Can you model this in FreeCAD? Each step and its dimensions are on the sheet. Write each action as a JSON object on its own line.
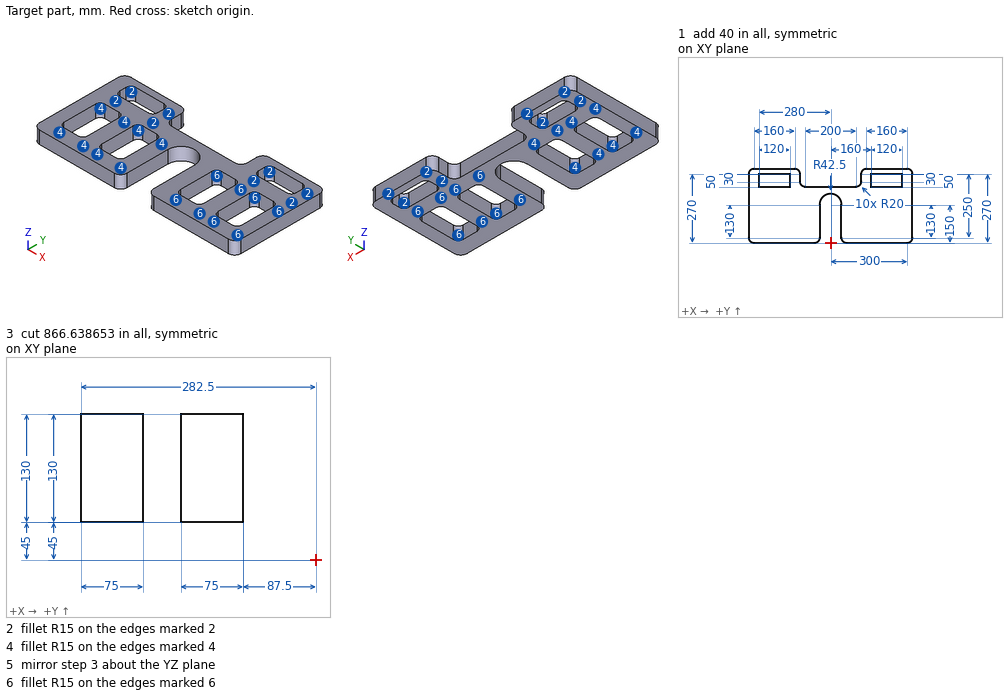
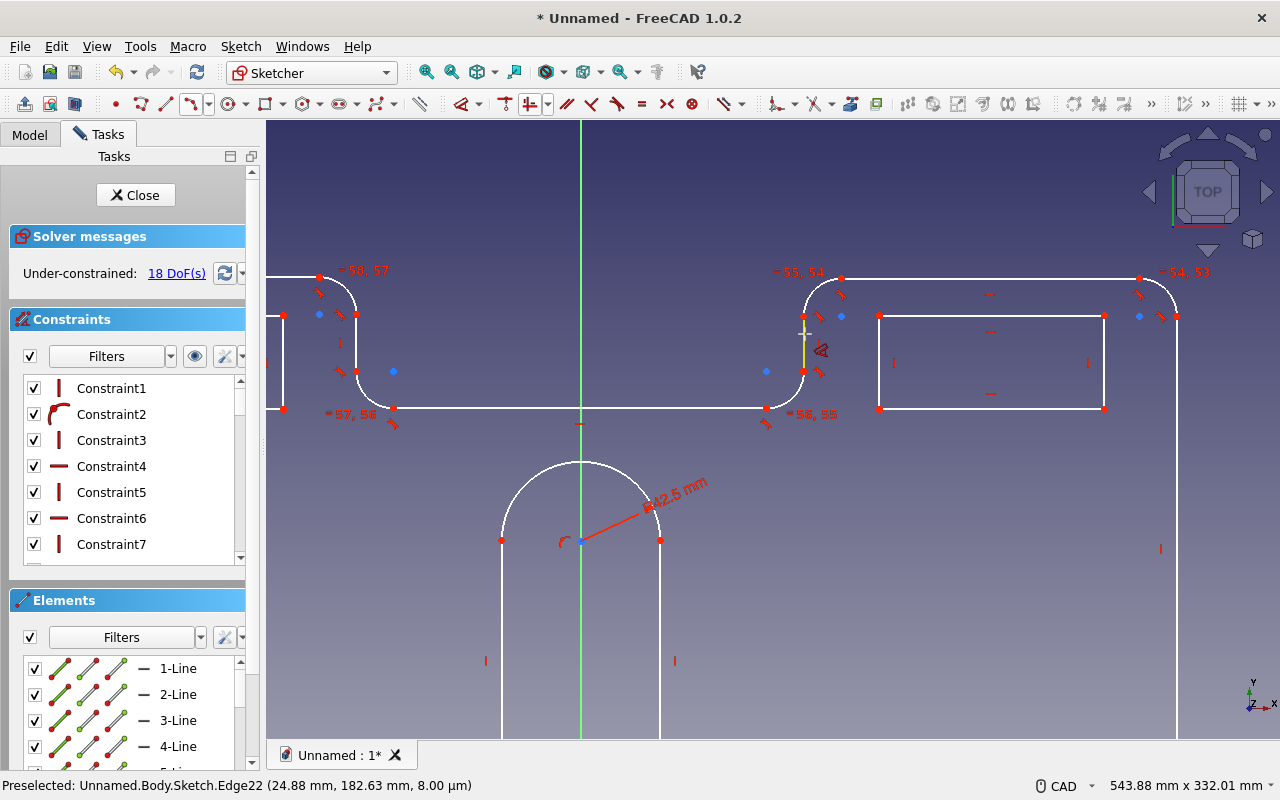
{"action": "left_click", "coordinate": [804, 333]}
{"action": "left_click", "coordinate": [838, 344]}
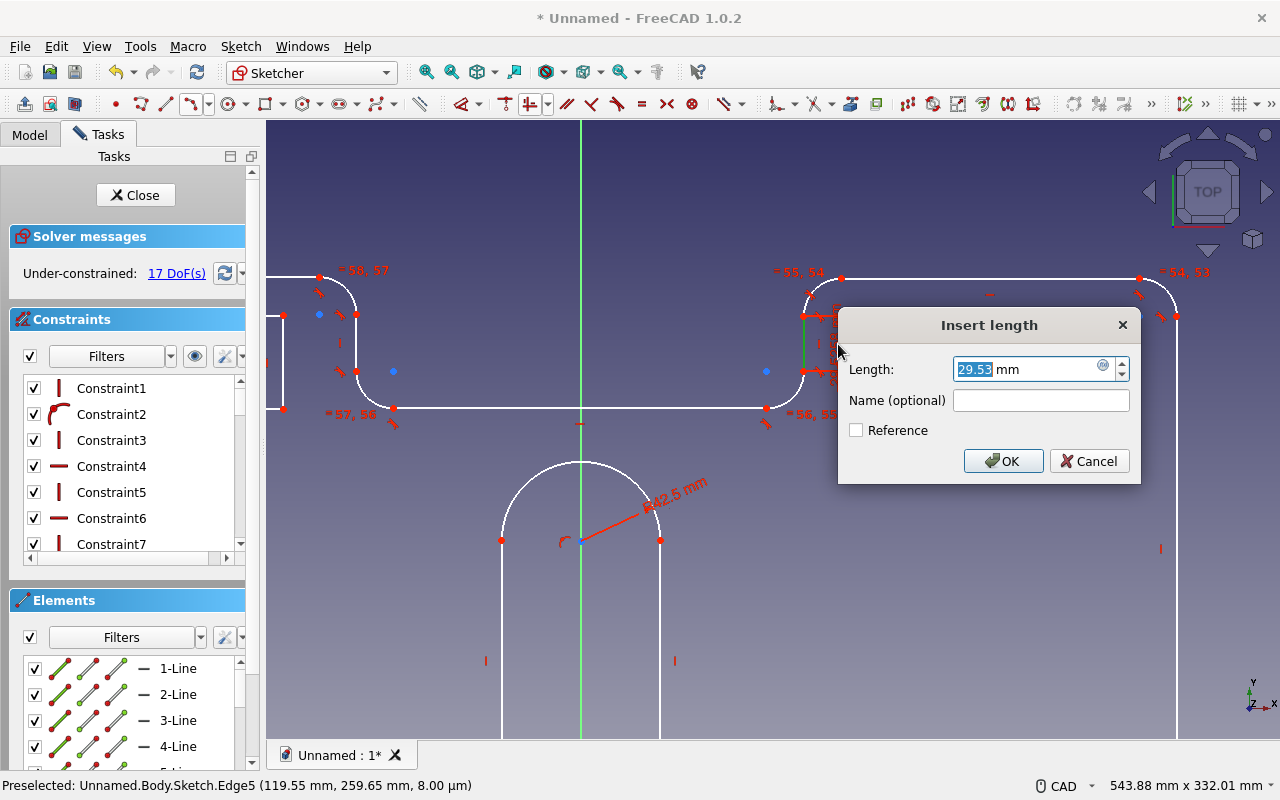
{"action": "type", "text": "30"}
{"action": "key", "text": "Return"}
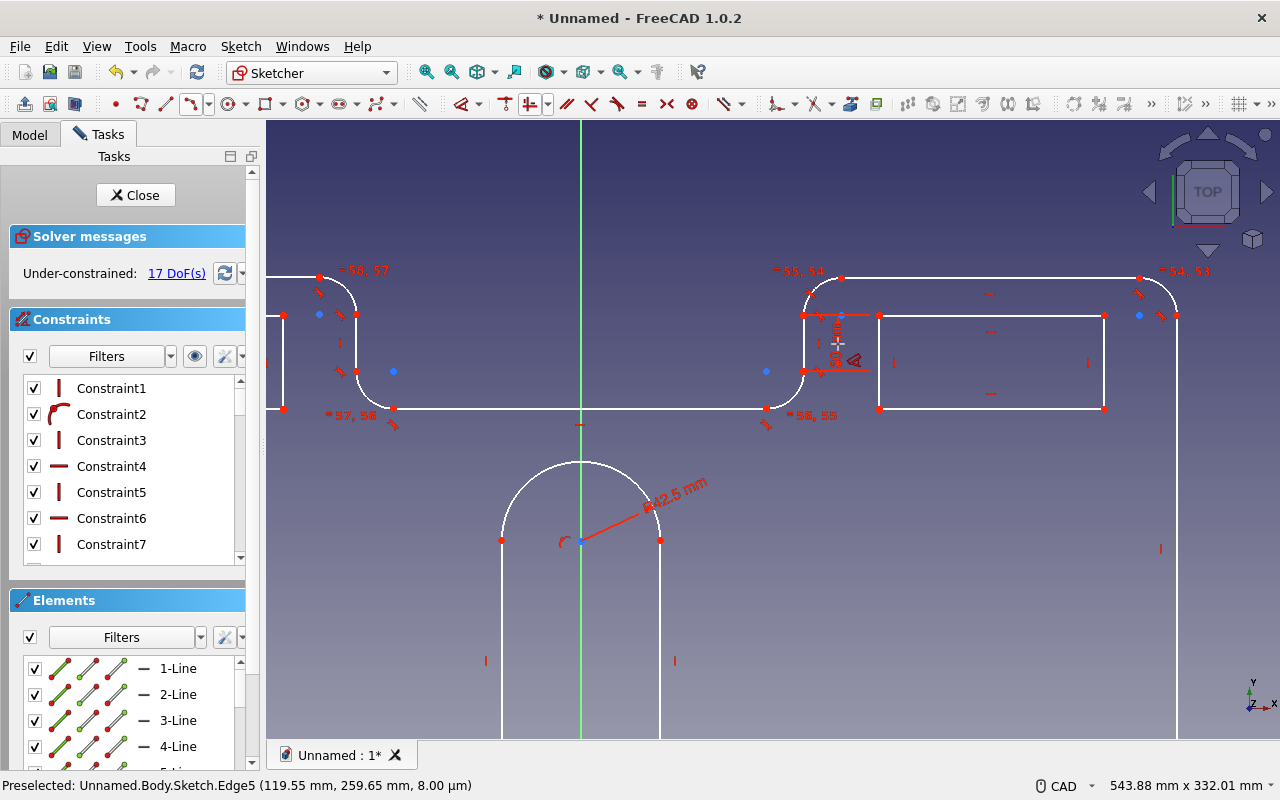
{"action": "left_click", "coordinate": [356, 354]}
{"action": "left_click", "coordinate": [322, 343]}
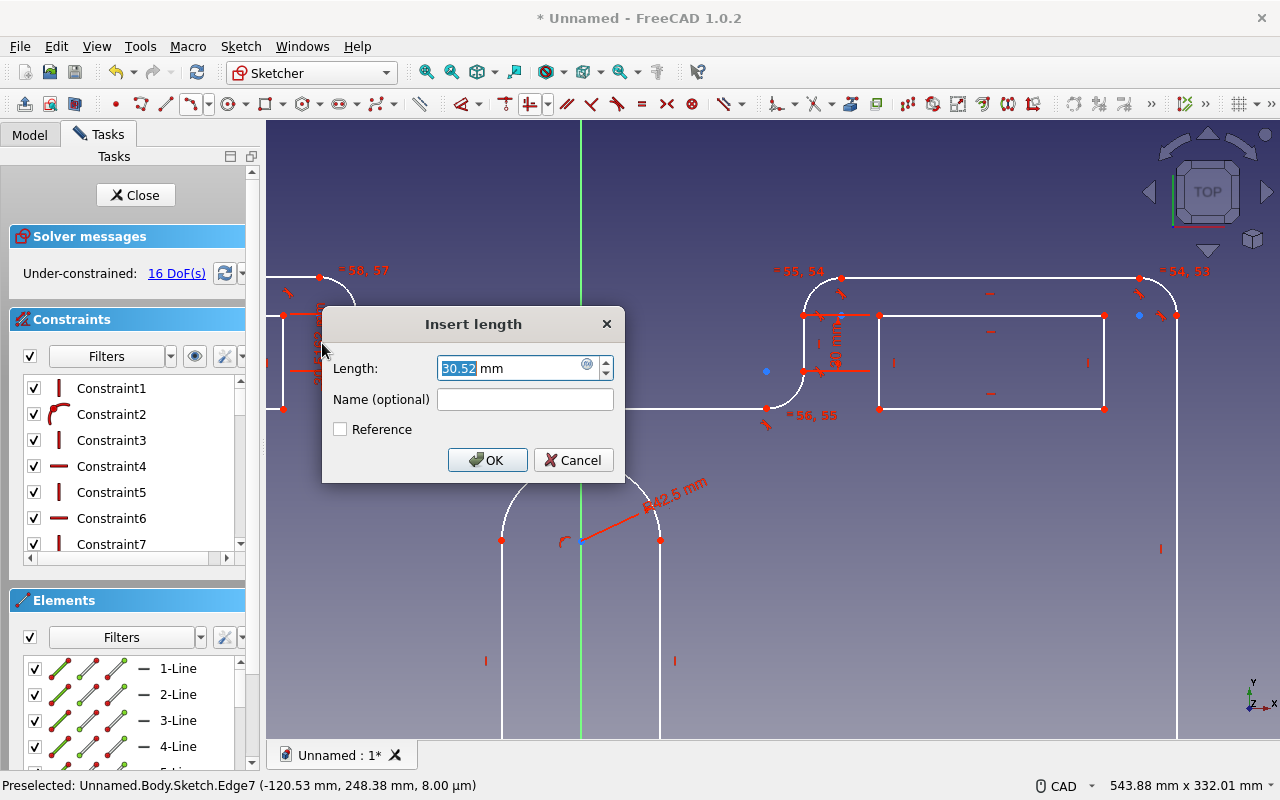
{"action": "type", "text": "30"}
{"action": "key", "text": "Return"}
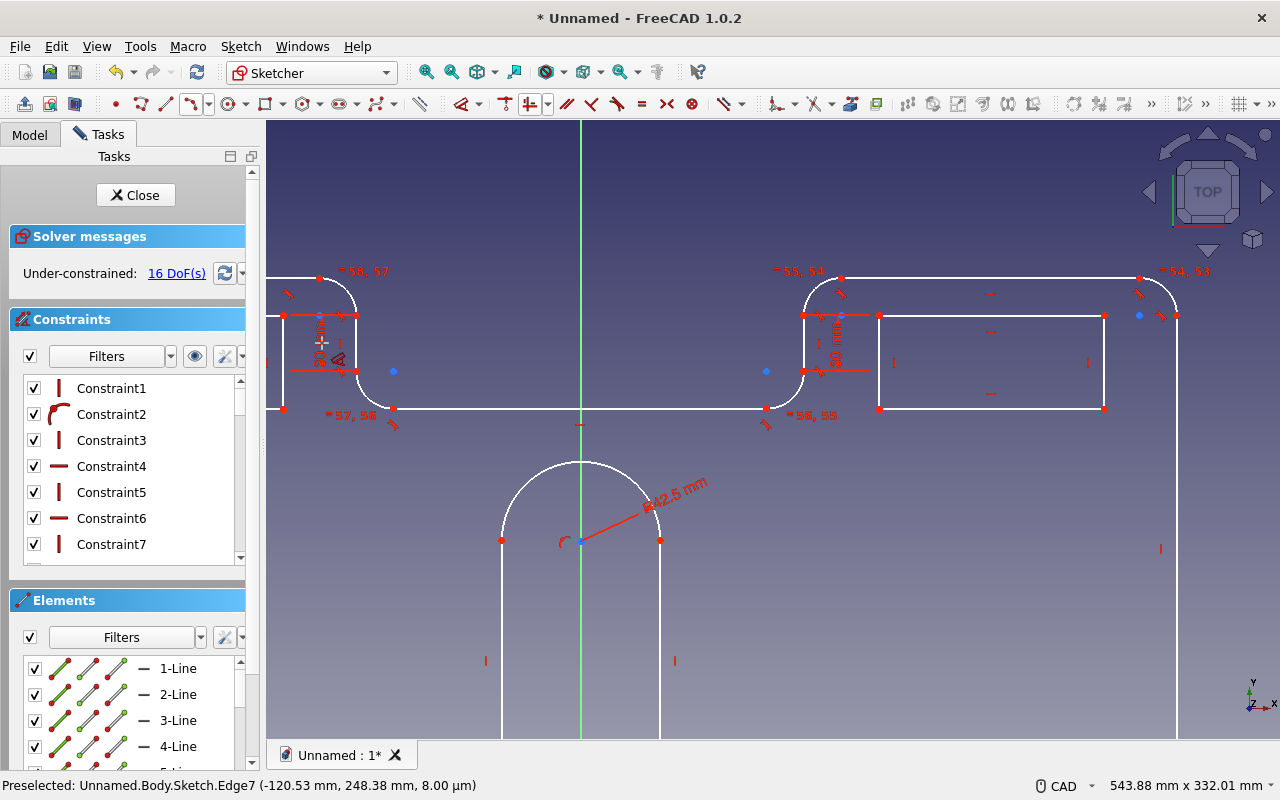
{"action": "scroll", "coordinate": [805, 333], "scroll_direction": "down", "scroll_amount": 4}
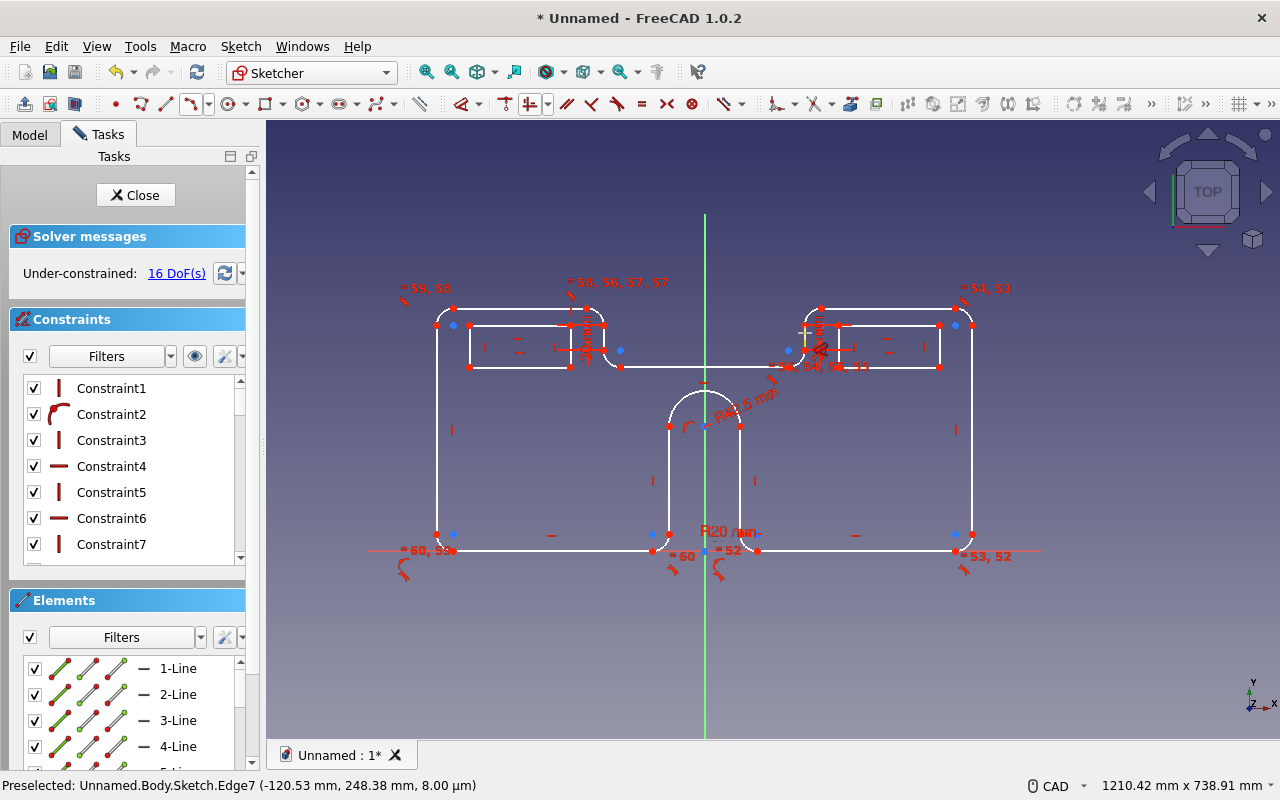
{"action": "left_click", "coordinate": [470, 338]}
{"action": "left_click", "coordinate": [504, 347]}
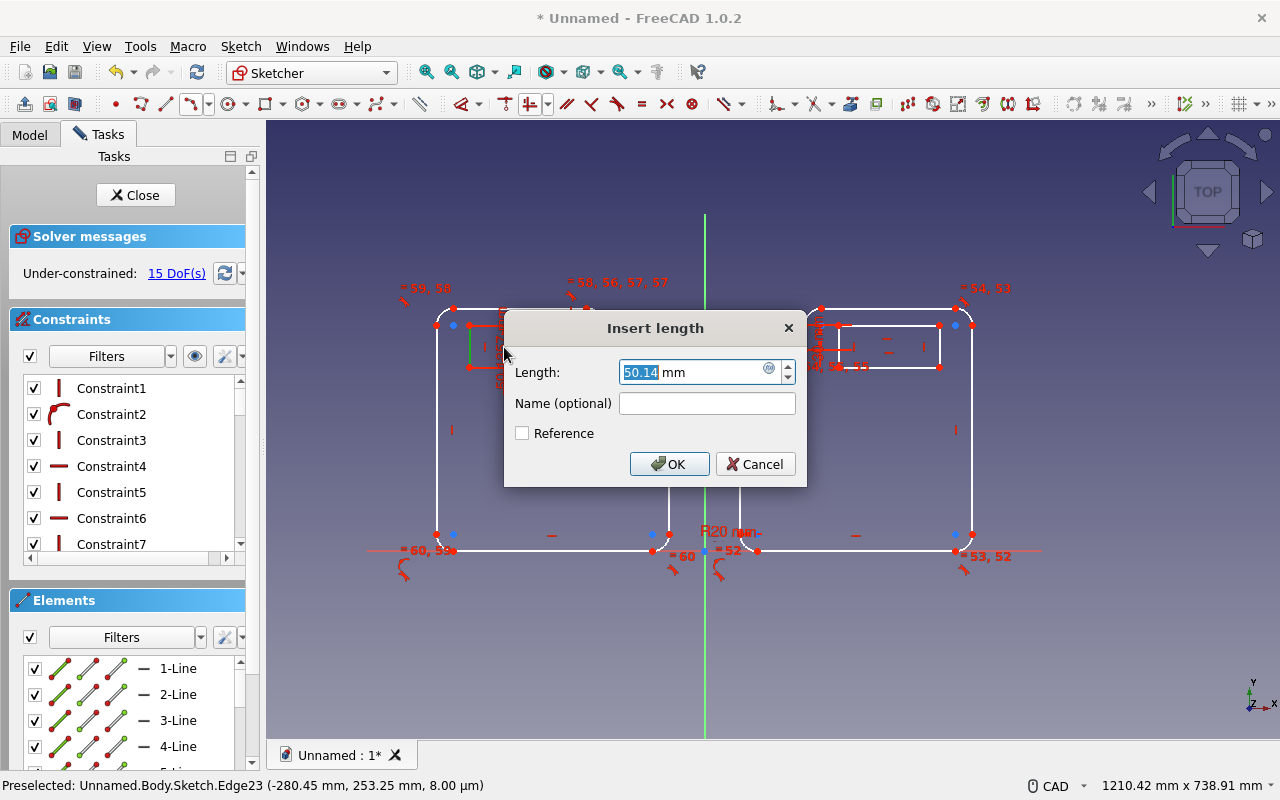
{"action": "type", "text": "50"}
{"action": "key", "text": "Return"}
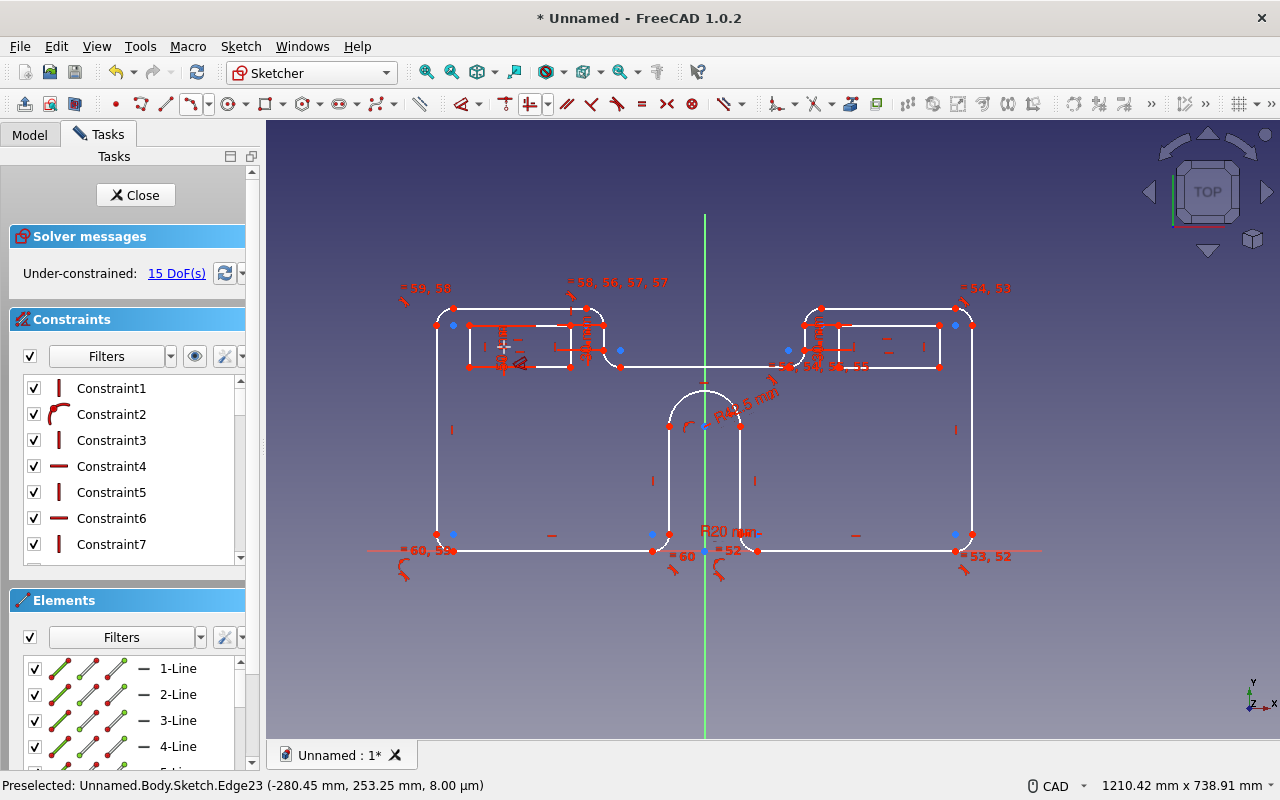
{"action": "left_click", "coordinate": [839, 338]}
{"action": "left_click", "coordinate": [897, 347]}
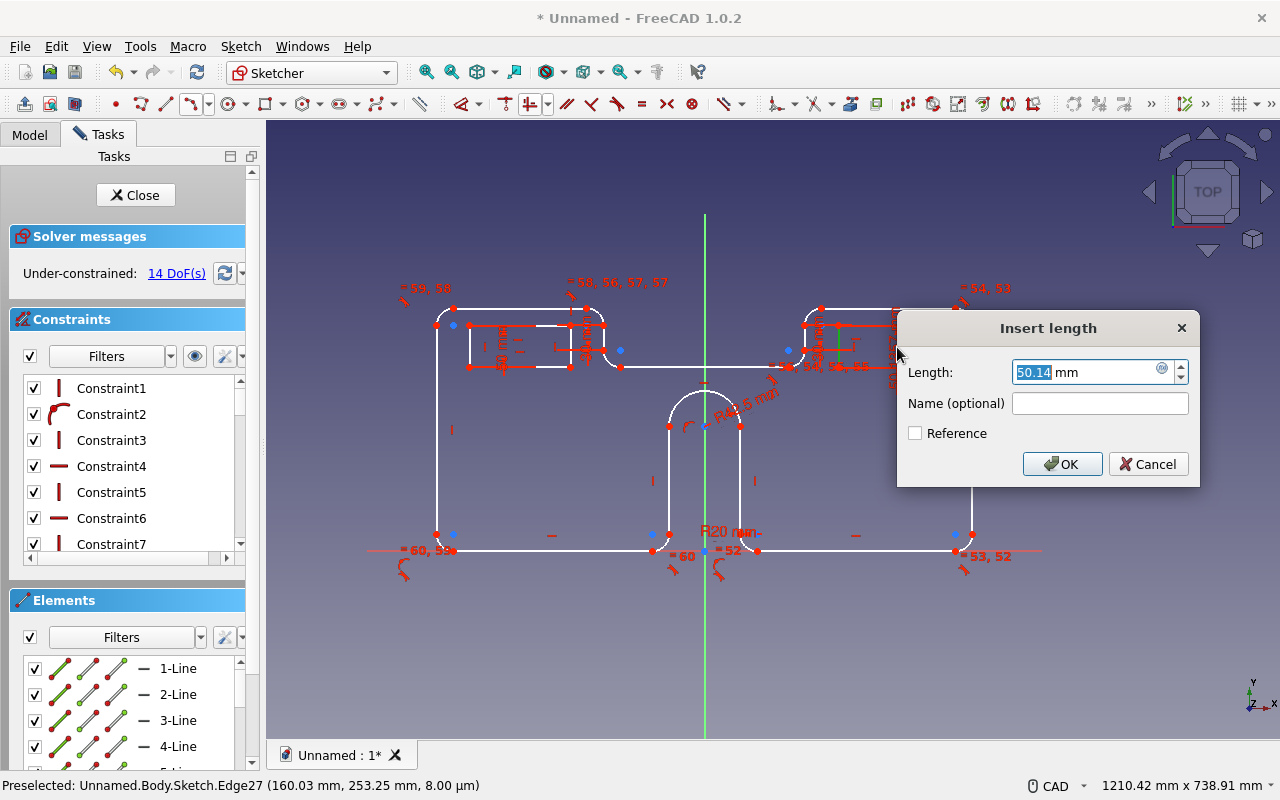
{"action": "type", "text": "50"}
{"action": "key", "text": "Return"}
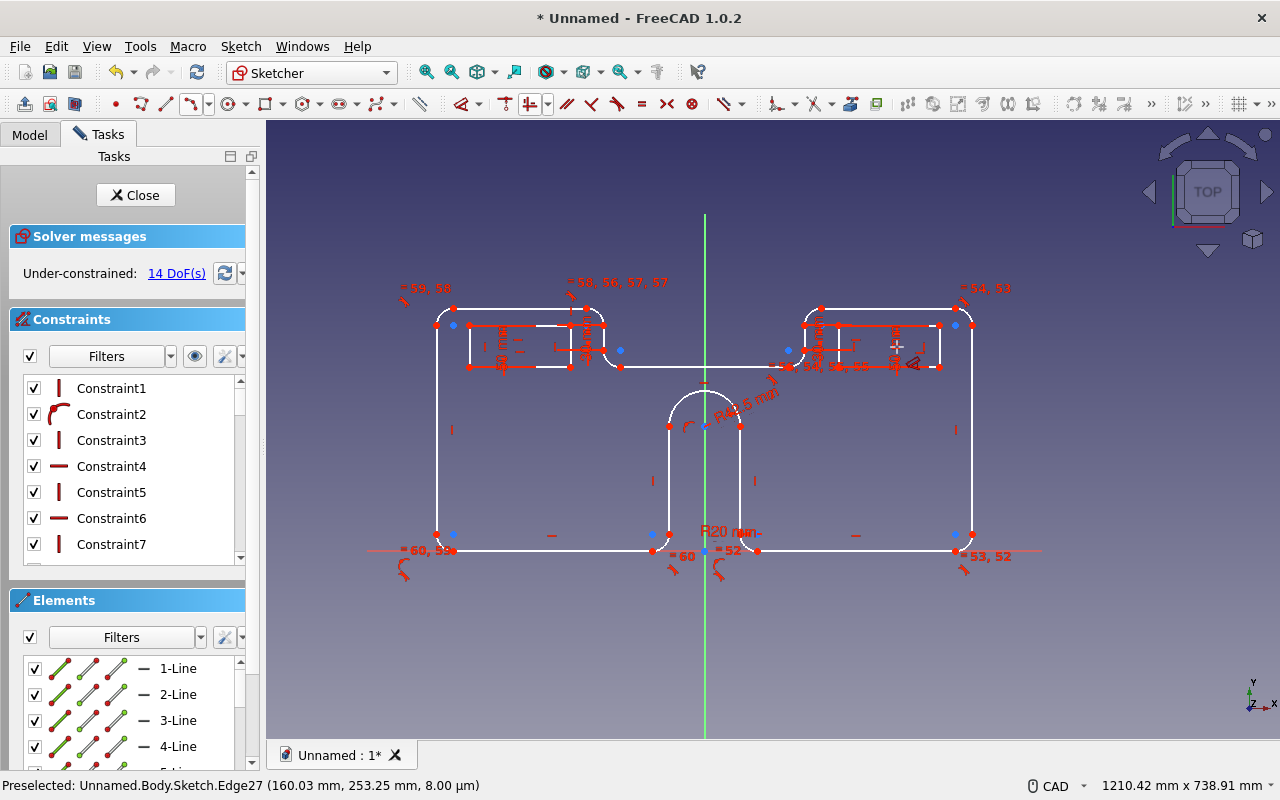
{"action": "left_click", "coordinate": [740, 459]}
{"action": "left_click", "coordinate": [774, 480]}